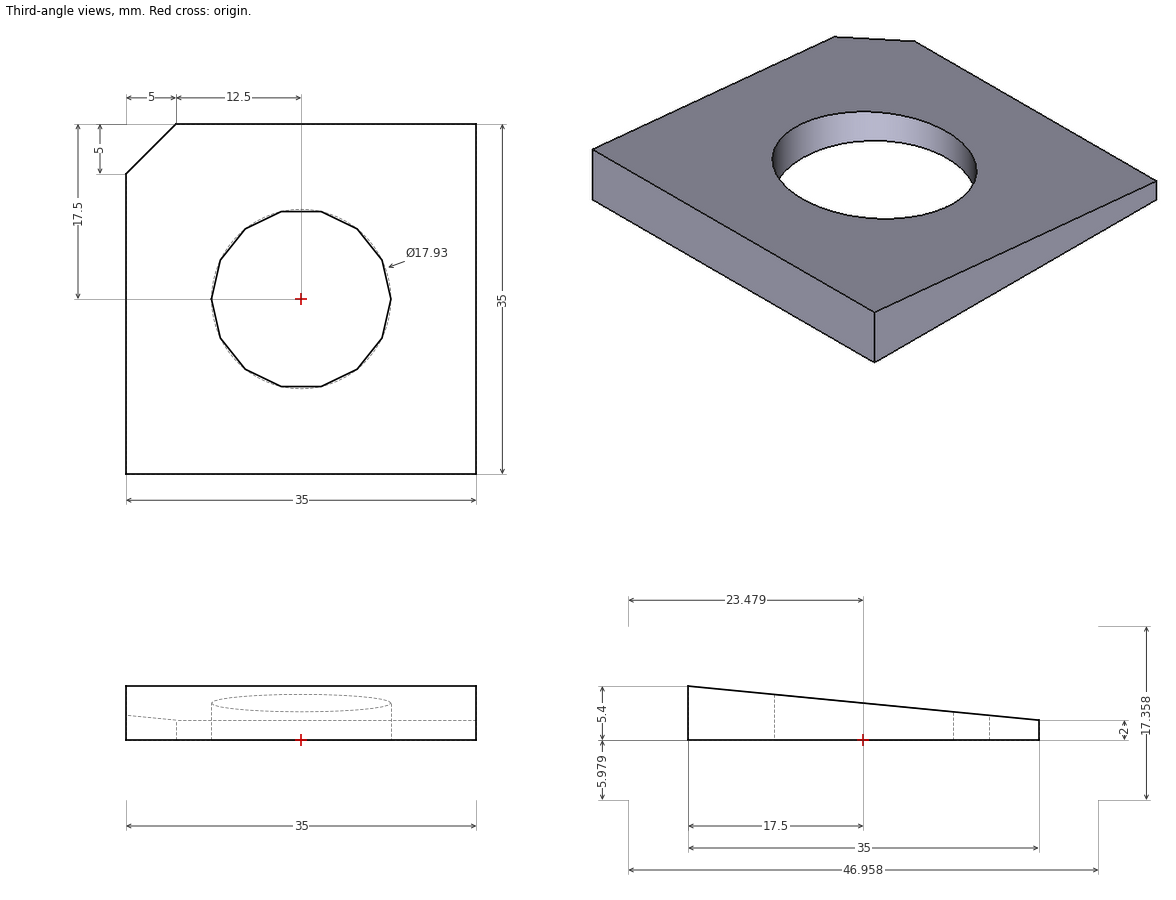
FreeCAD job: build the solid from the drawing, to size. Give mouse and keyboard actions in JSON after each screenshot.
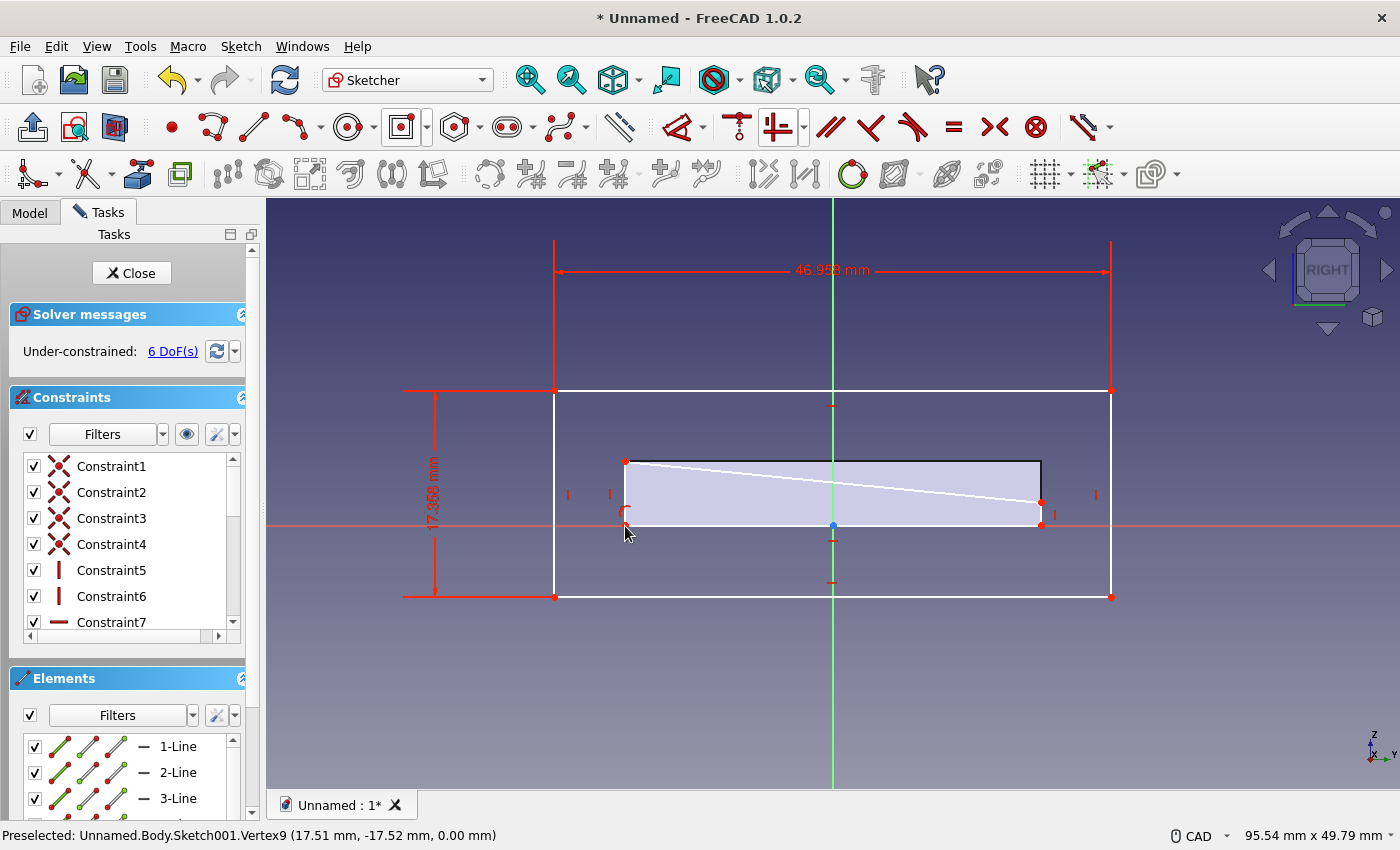
{"action": "scroll", "coordinate": [1041, 512], "scroll_direction": "up", "scroll_amount": 3}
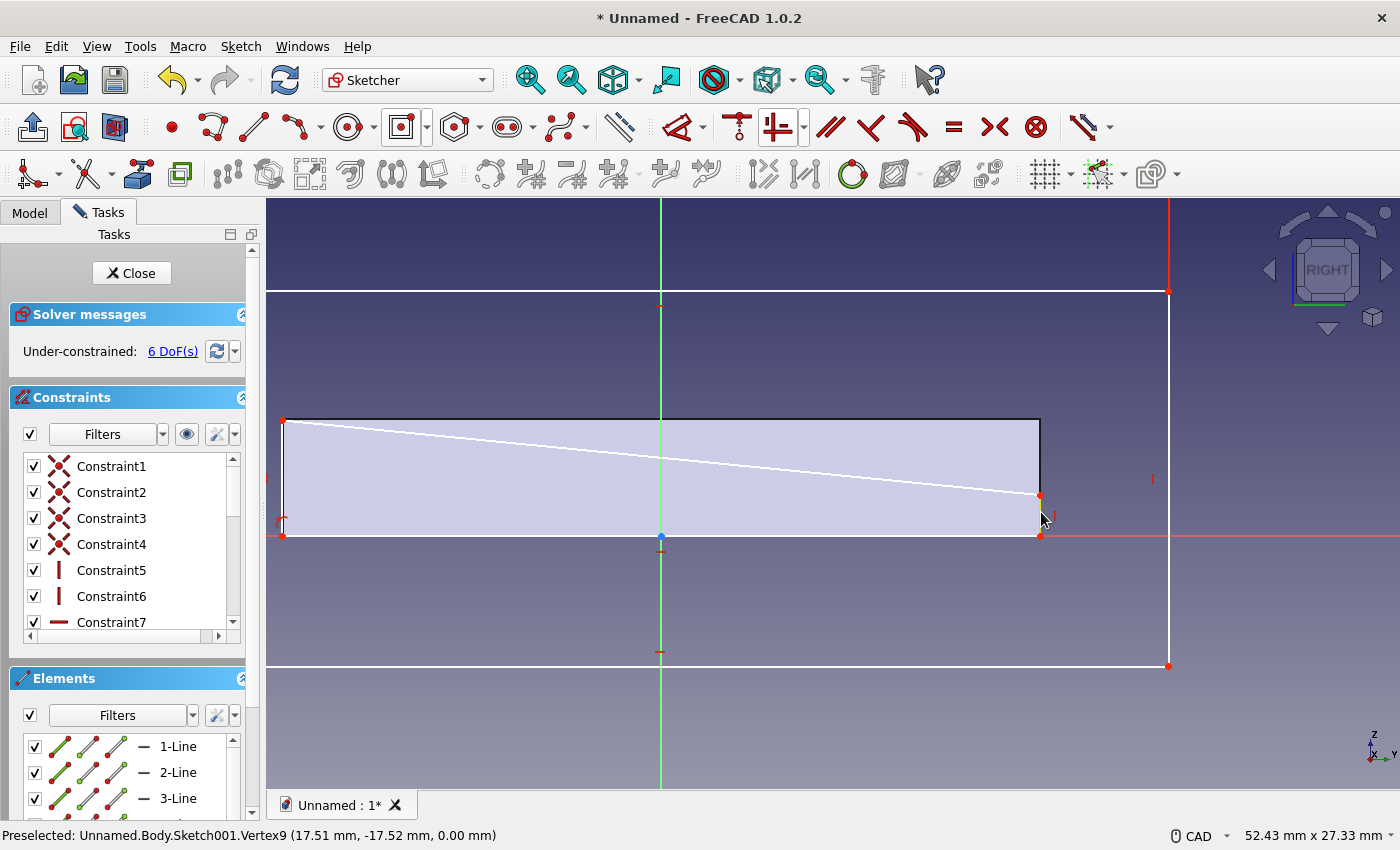
{"action": "left_click", "coordinate": [1040, 512]}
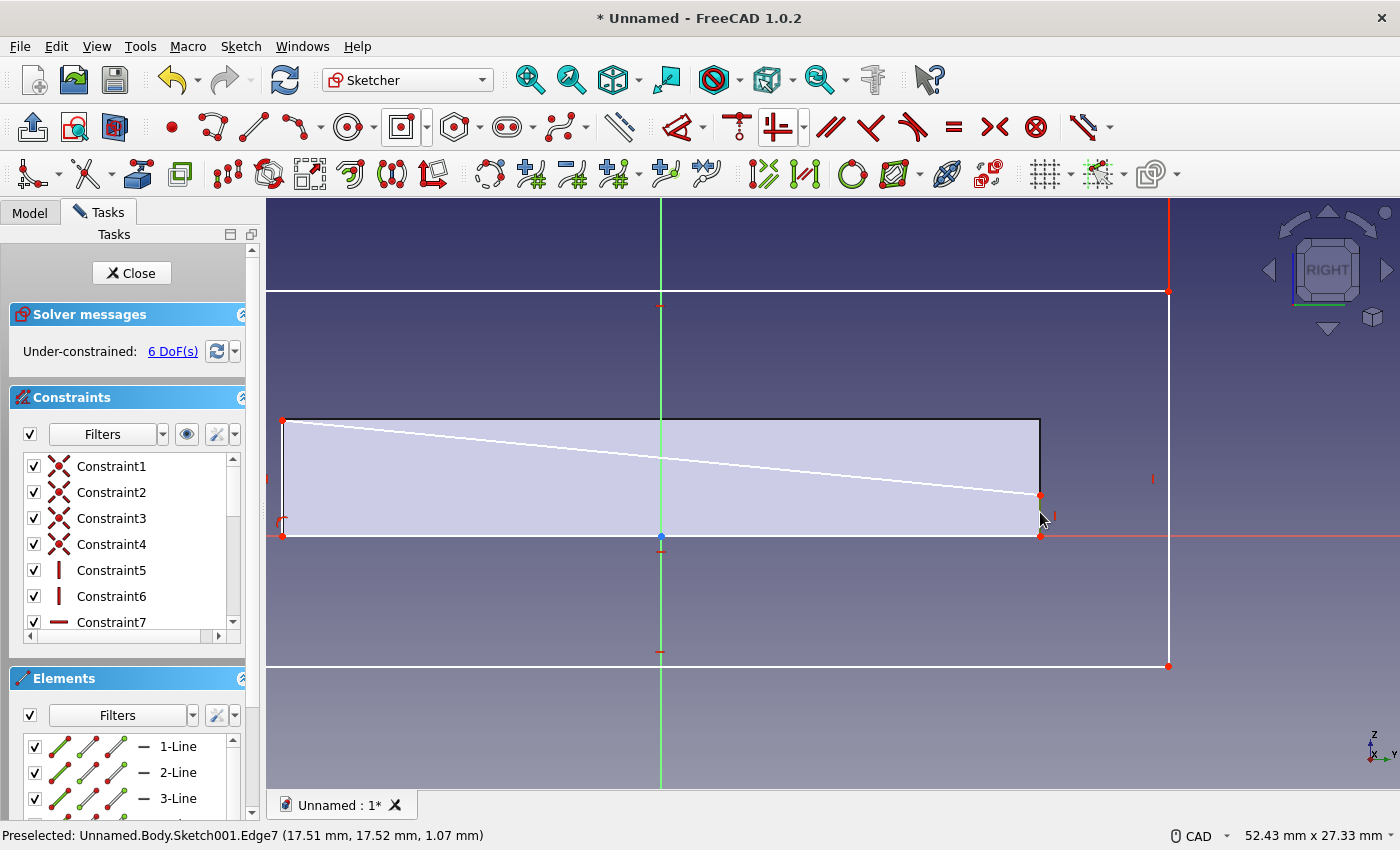
{"action": "key", "text": "i"}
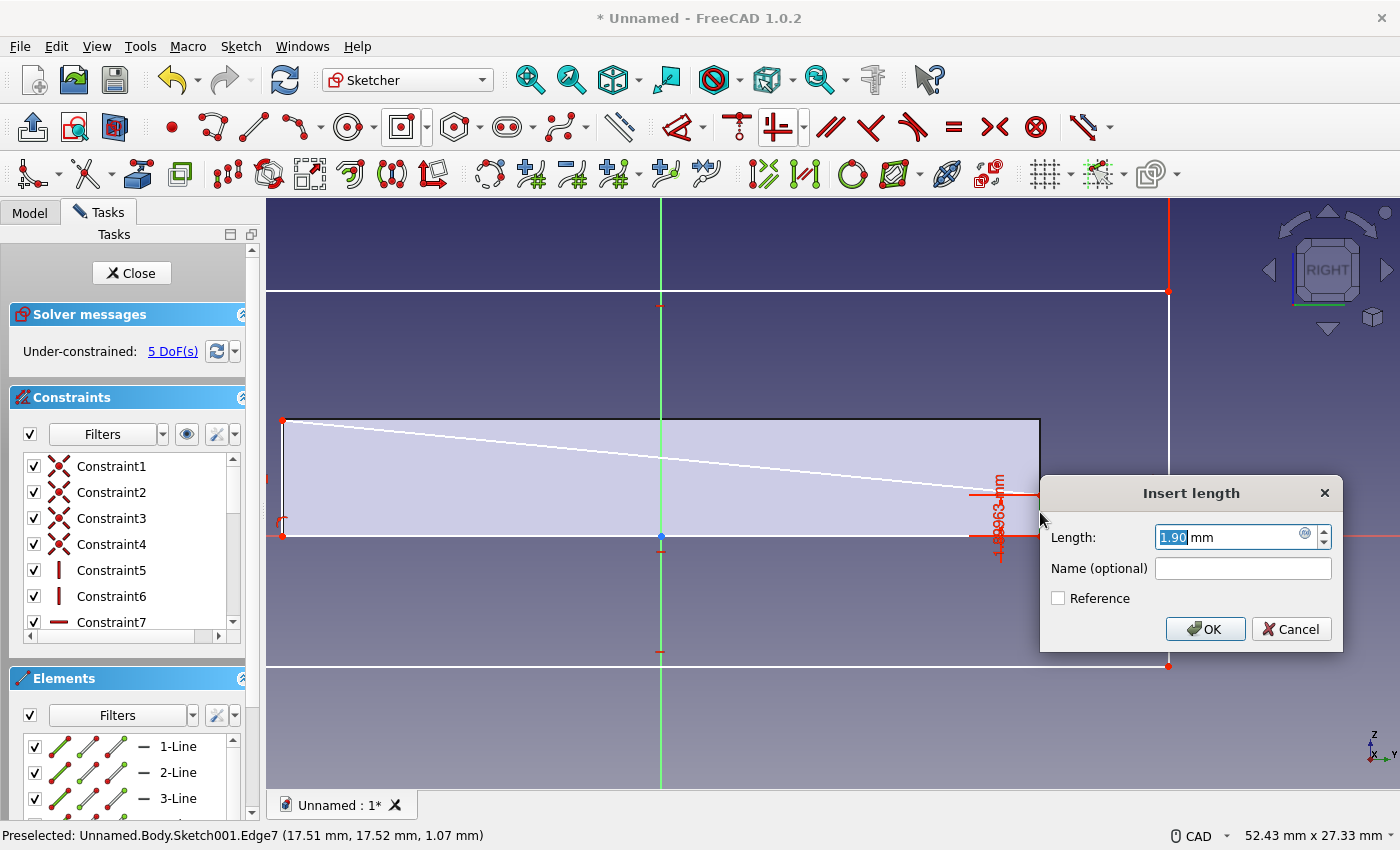
{"action": "type", "text": "2"}
{"action": "key", "text": "Return"}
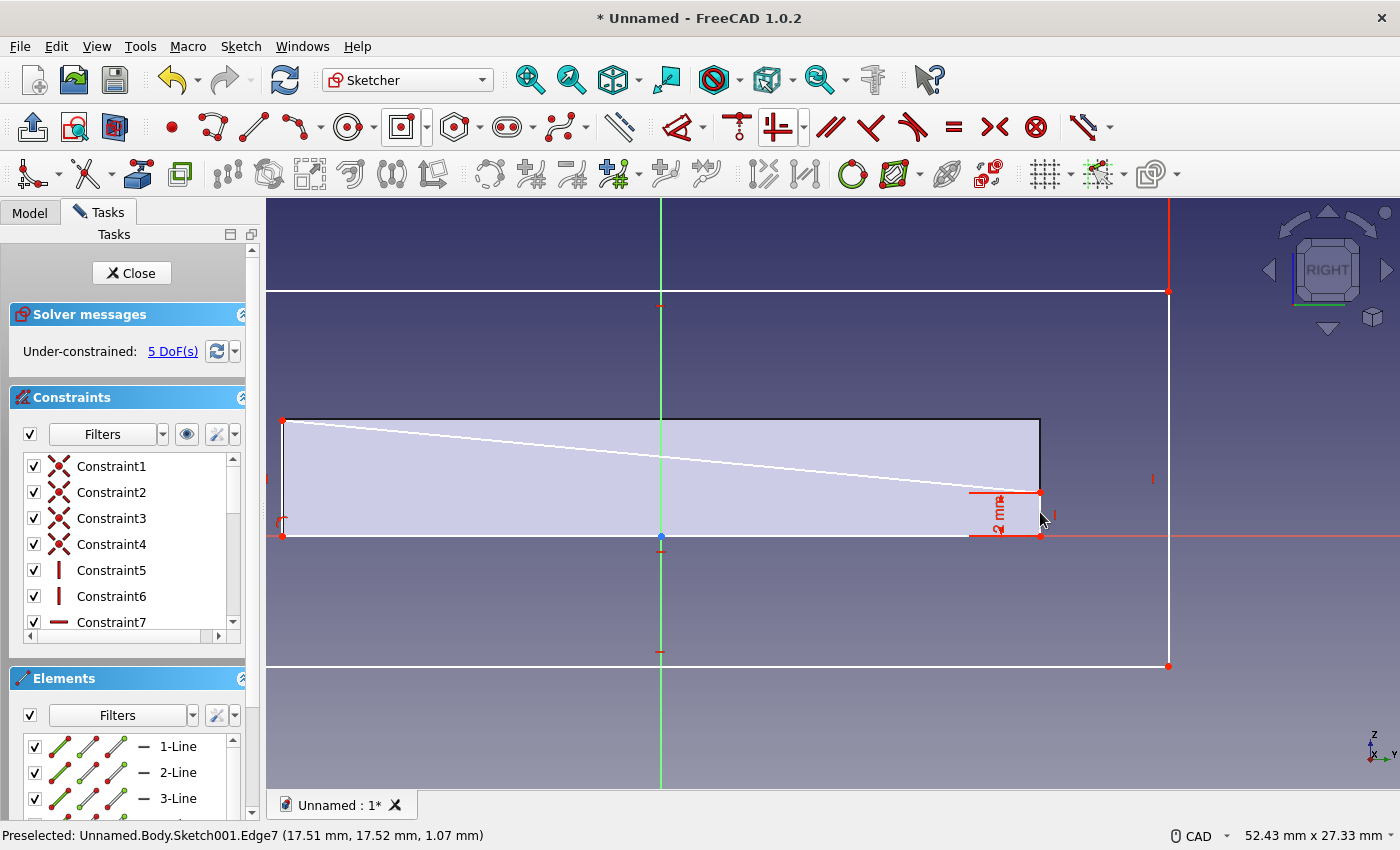
{"action": "left_click", "coordinate": [813, 536]}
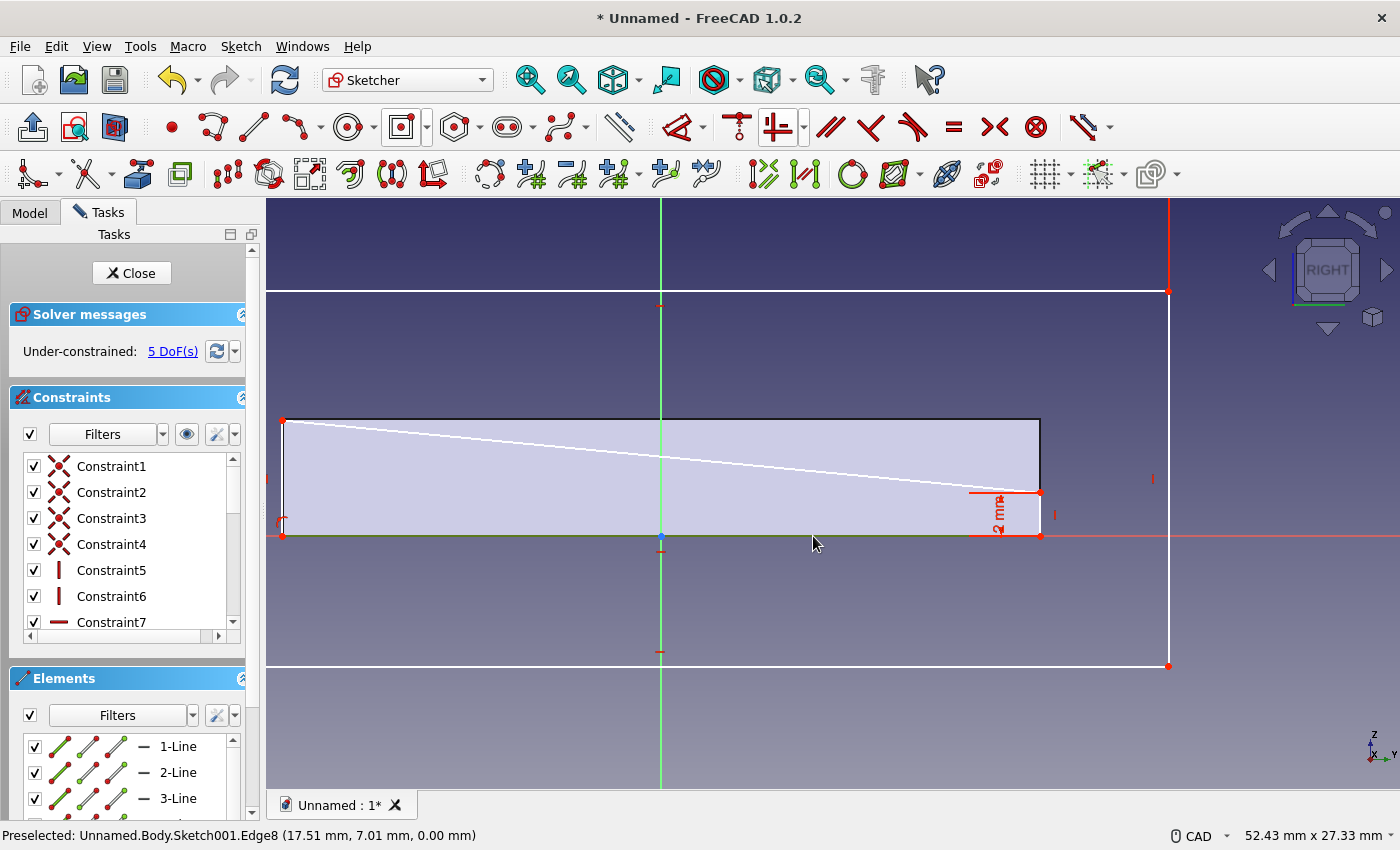
{"action": "key", "text": "l"}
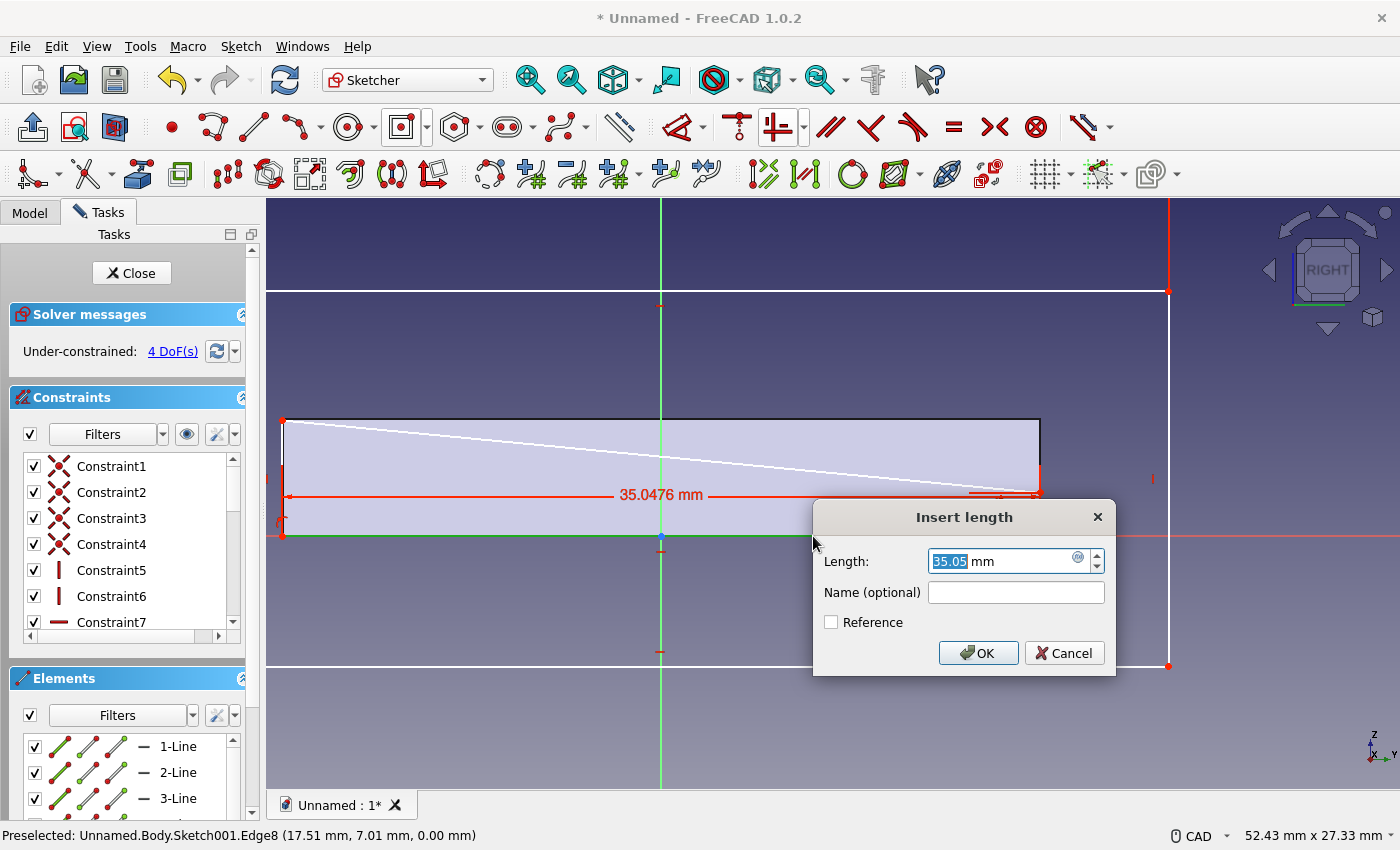
{"action": "type", "text": "35"}
{"action": "key", "text": "Return"}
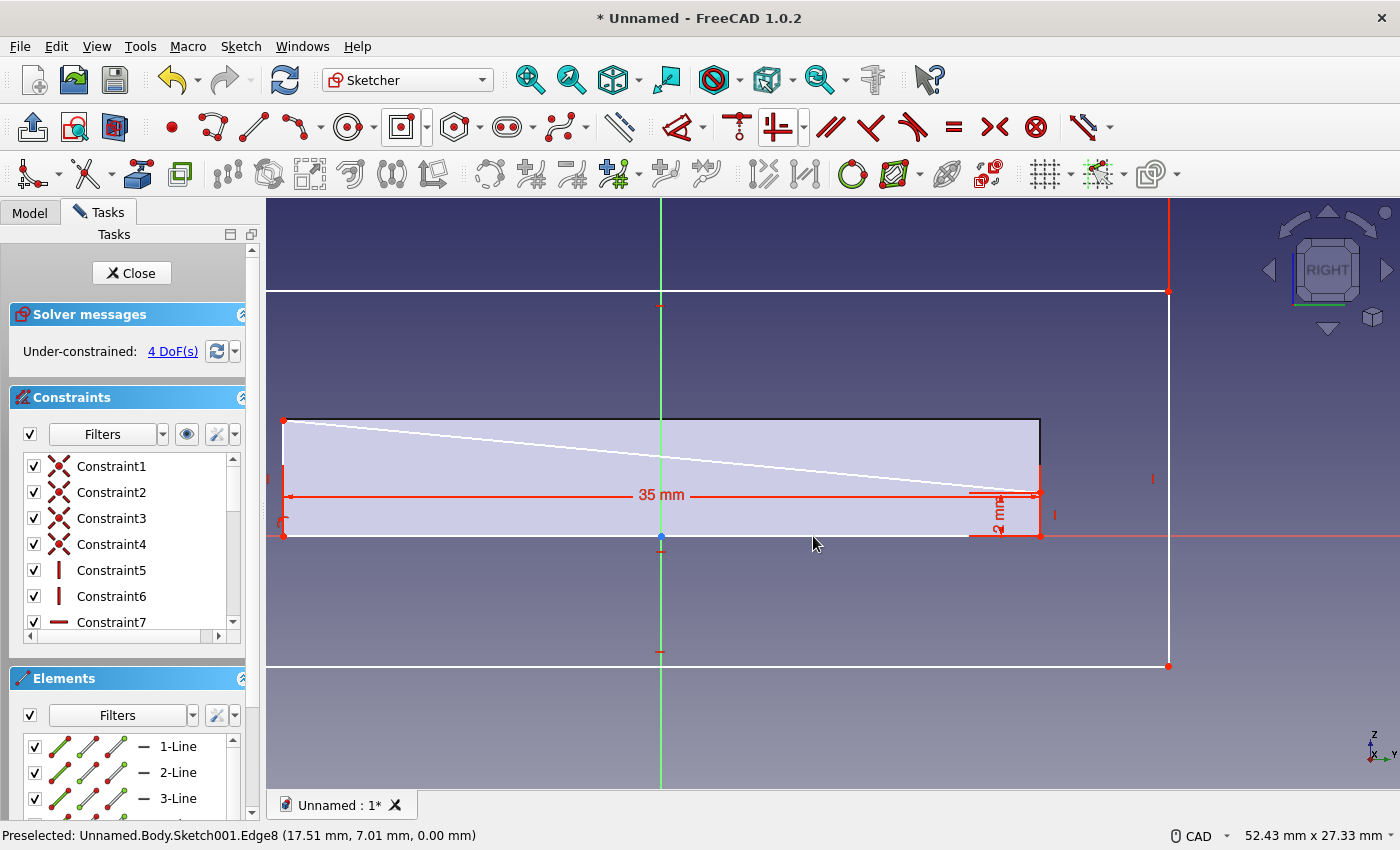
{"action": "scroll", "coordinate": [974, 525], "scroll_direction": "down", "scroll_amount": 2}